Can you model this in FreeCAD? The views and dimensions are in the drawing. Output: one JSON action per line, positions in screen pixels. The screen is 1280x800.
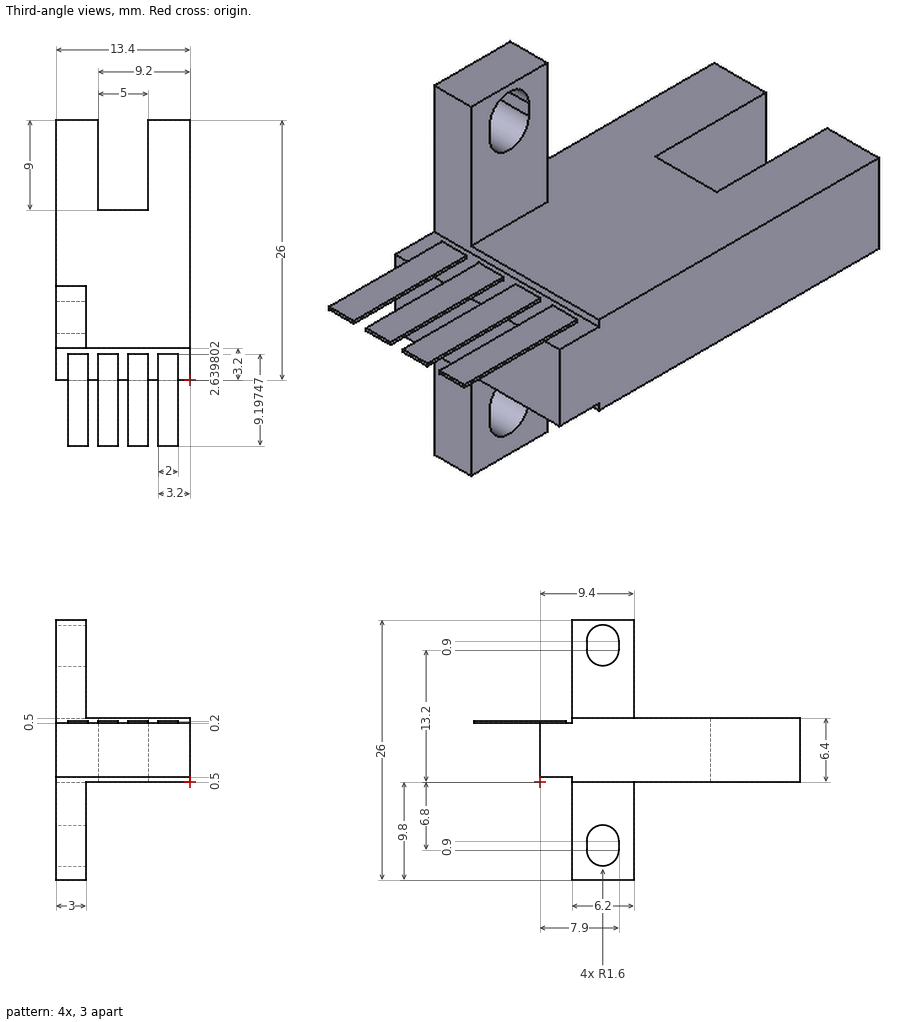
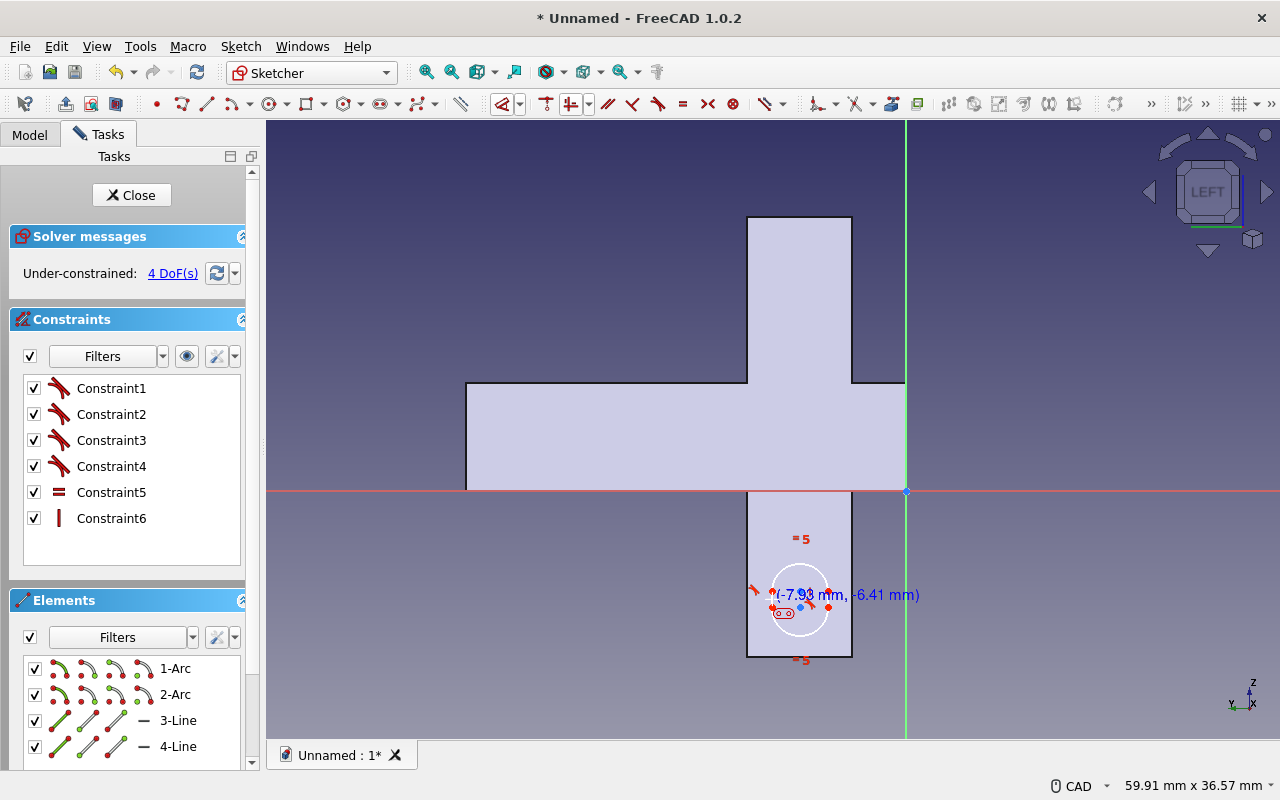
{"action": "left_click", "coordinate": [800, 268]}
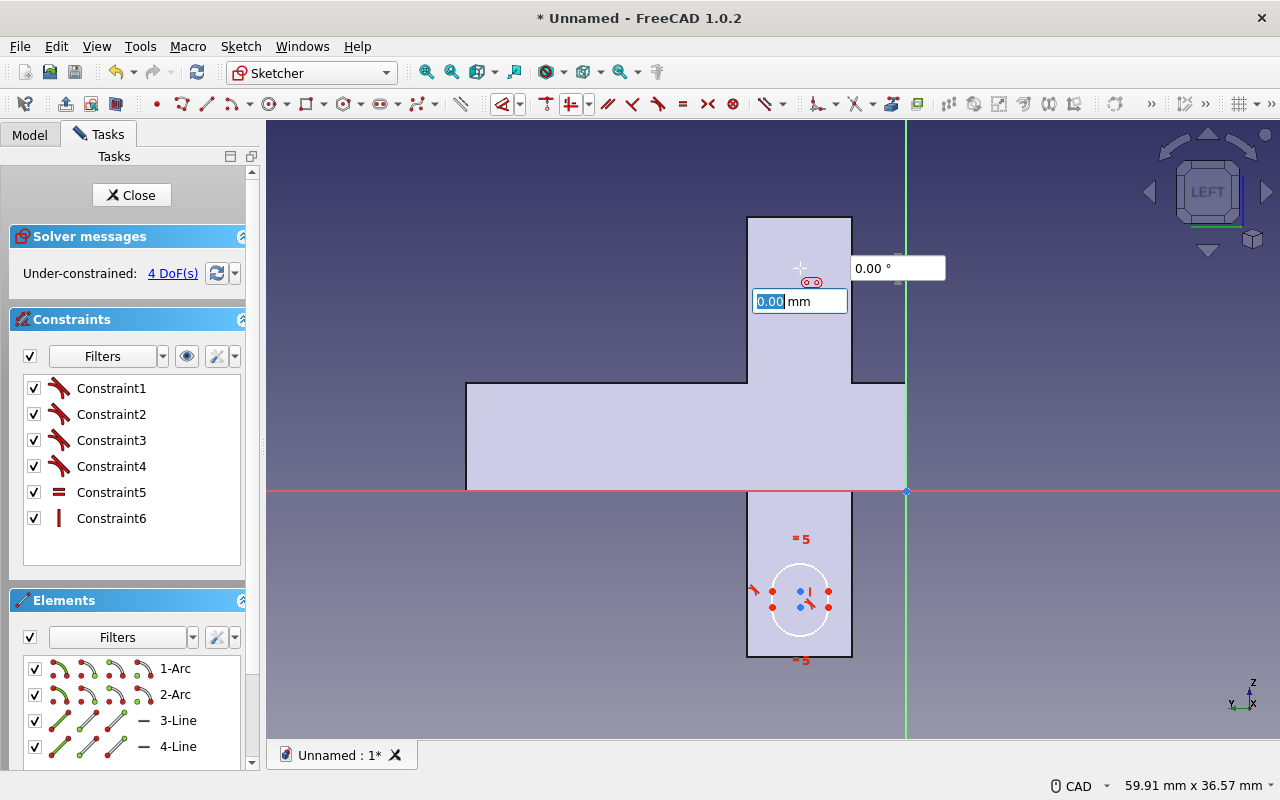
{"action": "left_click", "coordinate": [800, 253]}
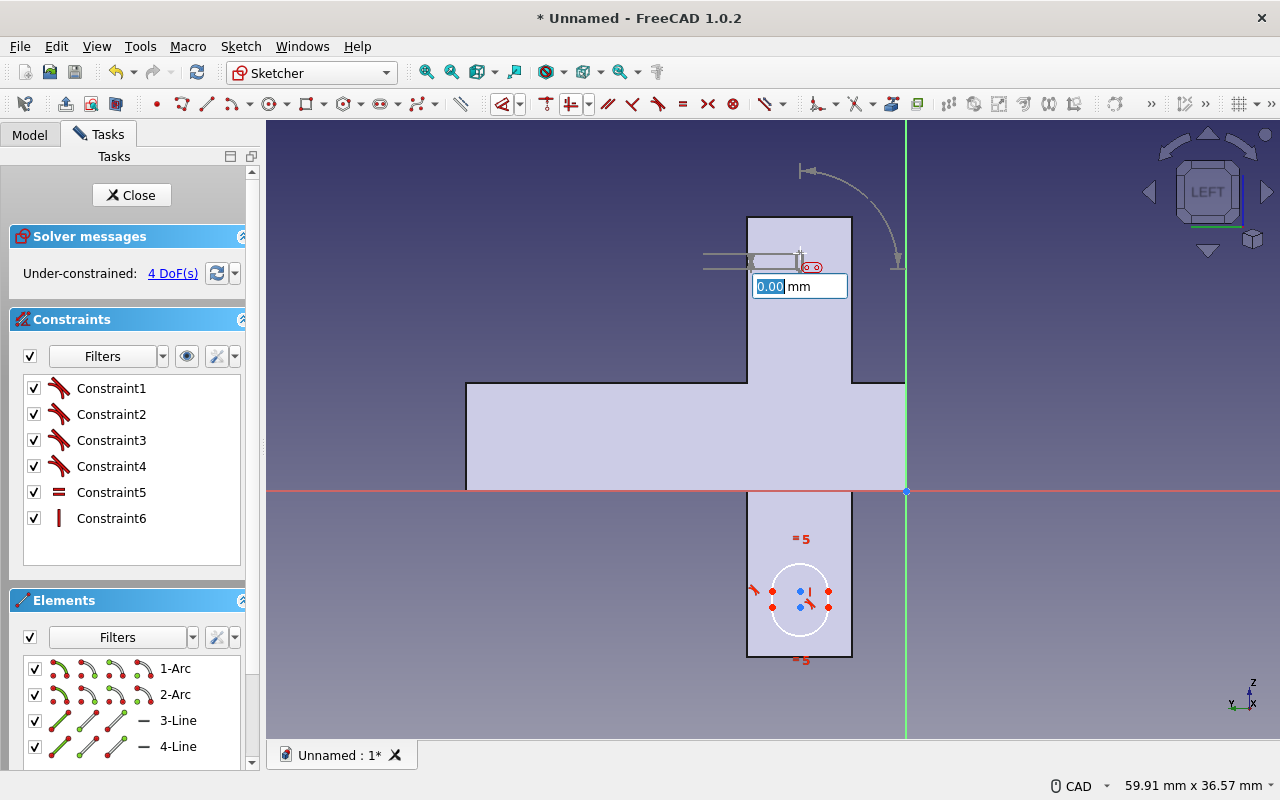
{"action": "left_click", "coordinate": [772, 260]}
{"action": "key", "text": "Escape"}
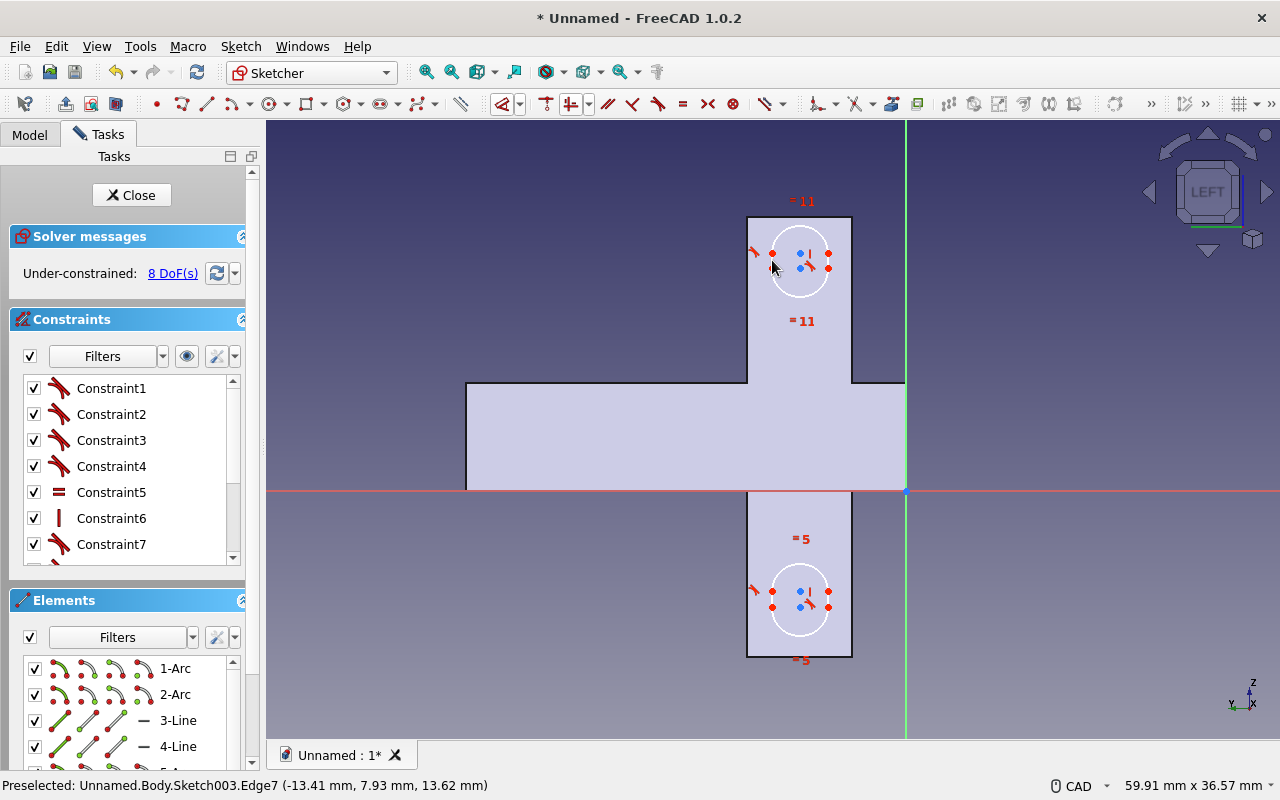
{"action": "left_click", "coordinate": [784, 631]}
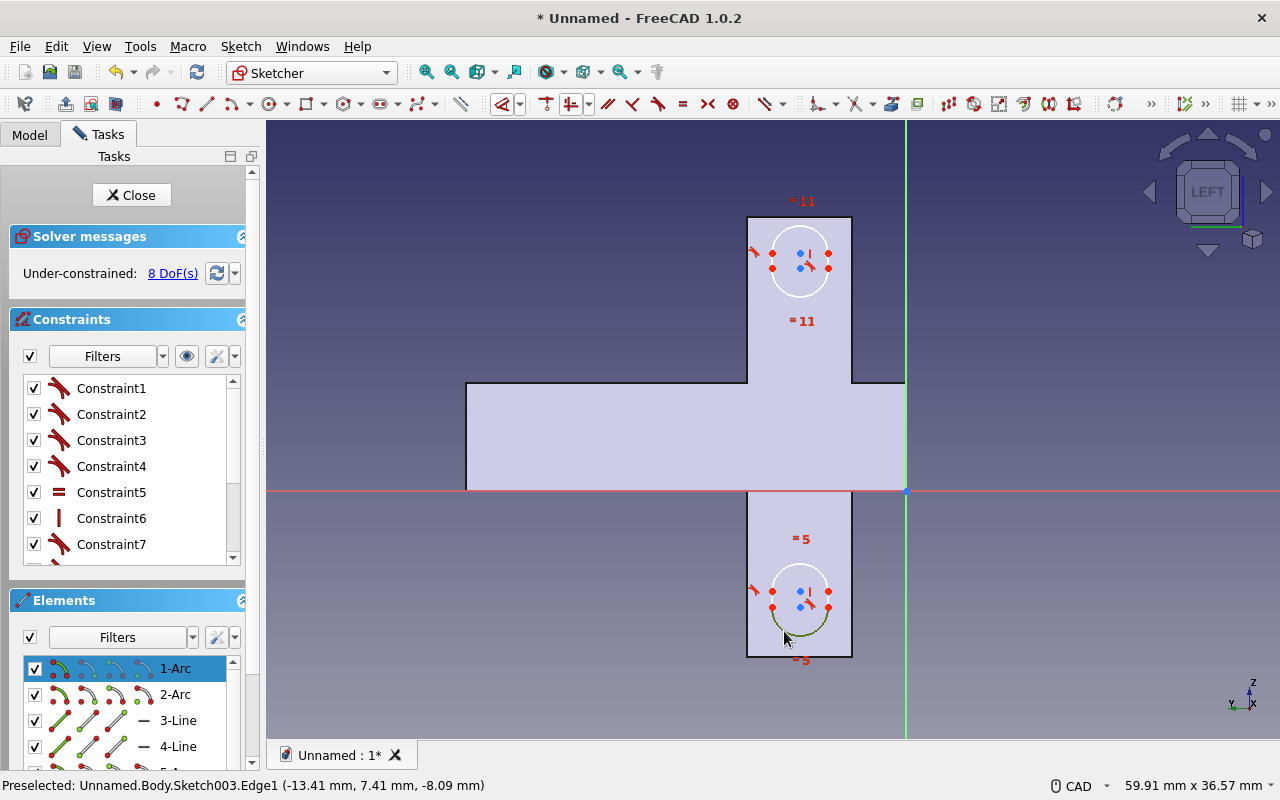
{"action": "left_click", "coordinate": [784, 292]}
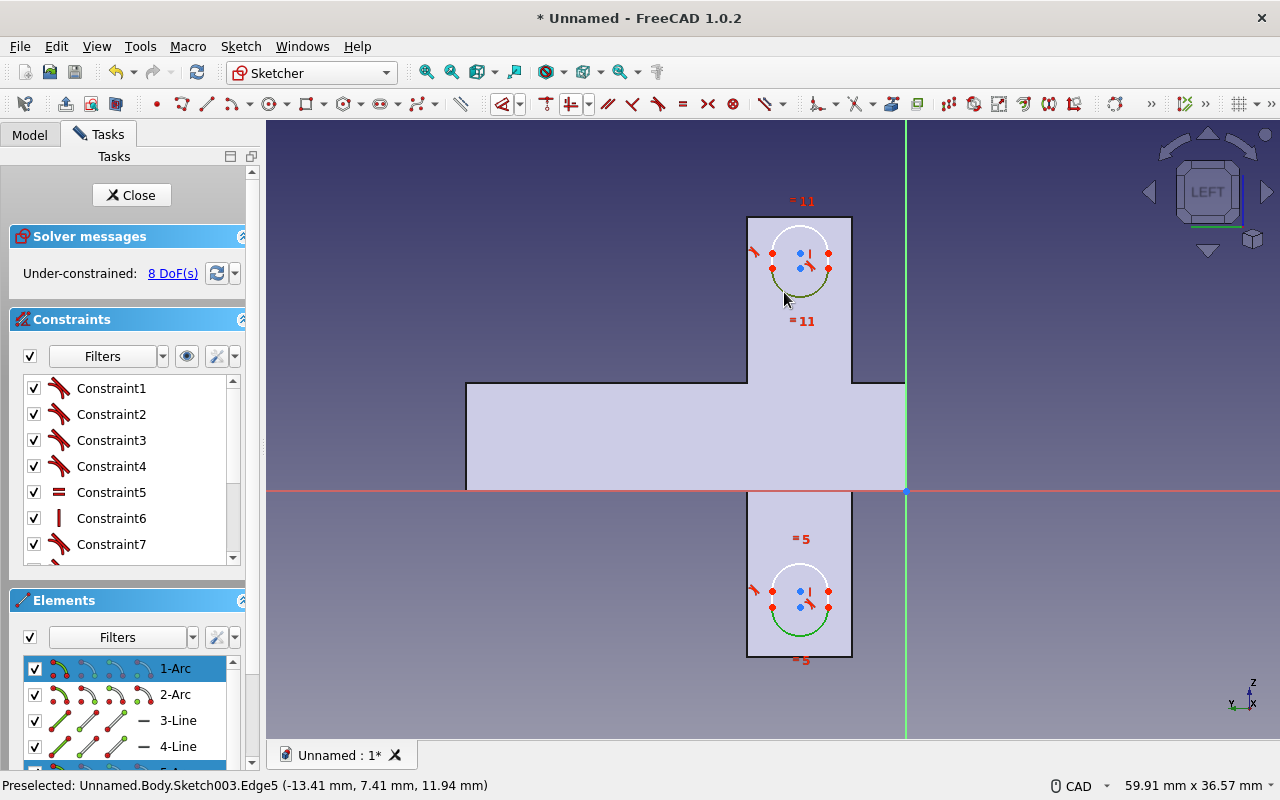
{"action": "left_click", "coordinate": [683, 104]}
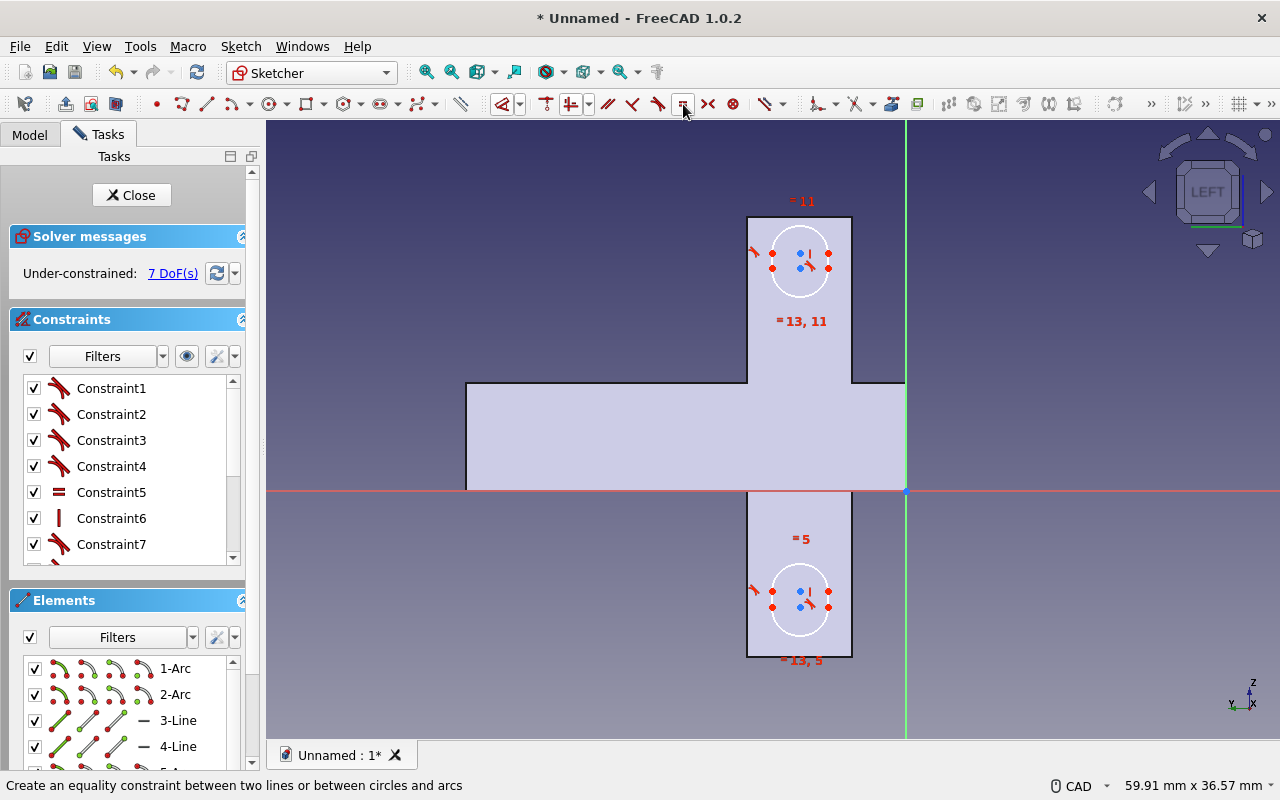
{"action": "scroll", "coordinate": [784, 631], "scroll_direction": "up", "scroll_amount": 2}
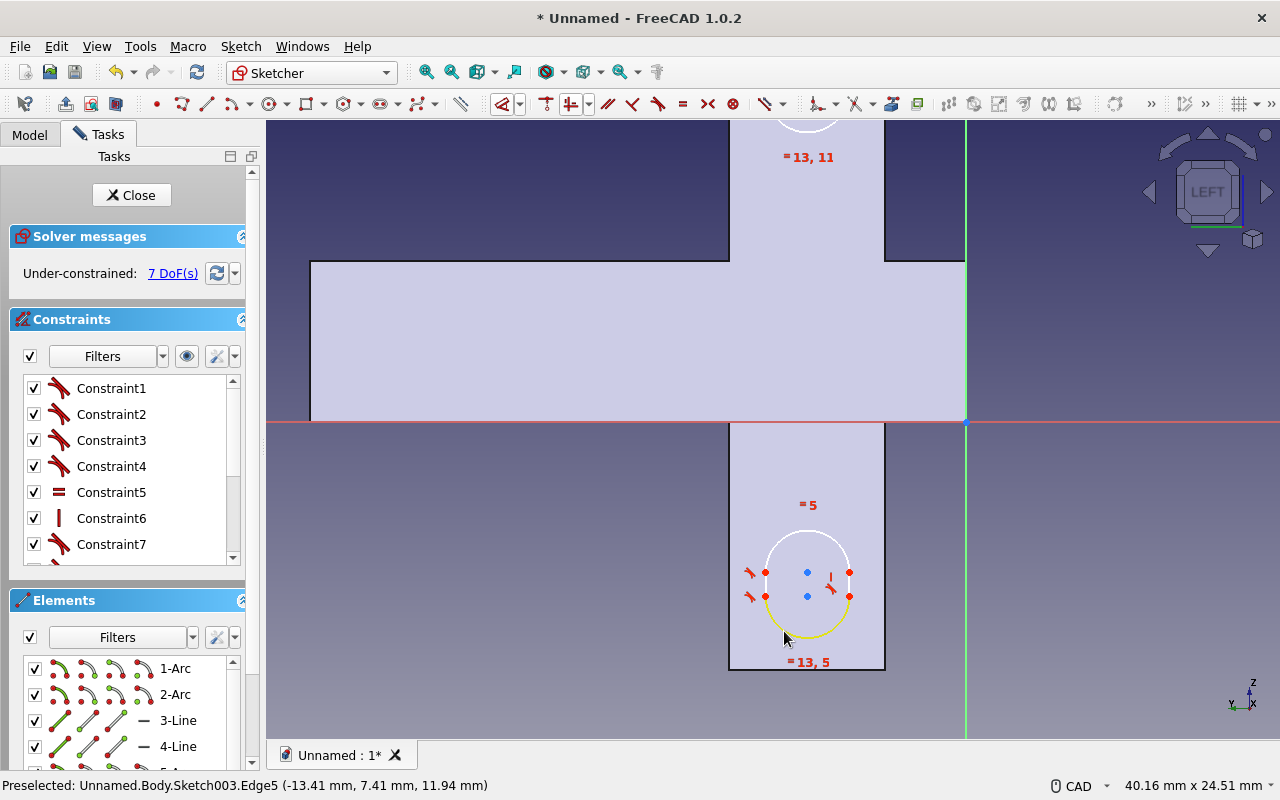
{"action": "left_click", "coordinate": [783, 630]}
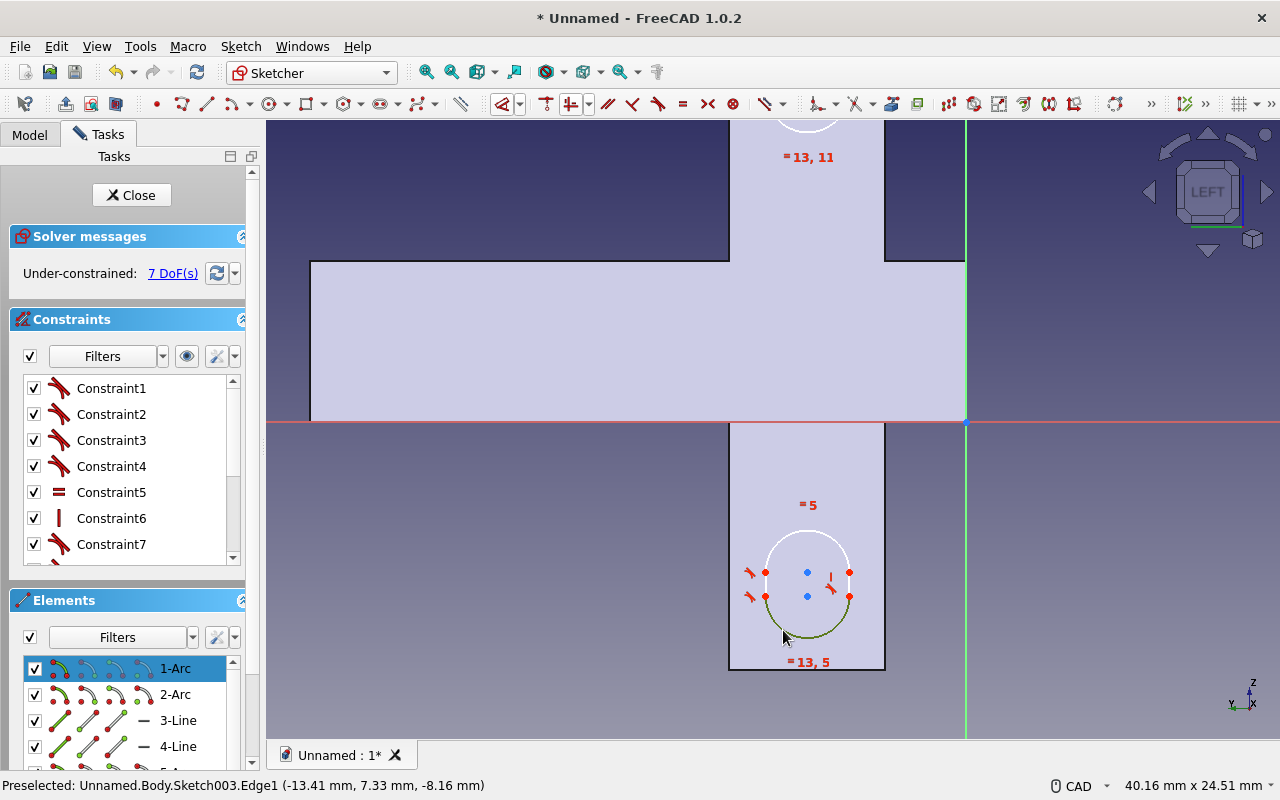
{"action": "left_click", "coordinate": [520, 104]}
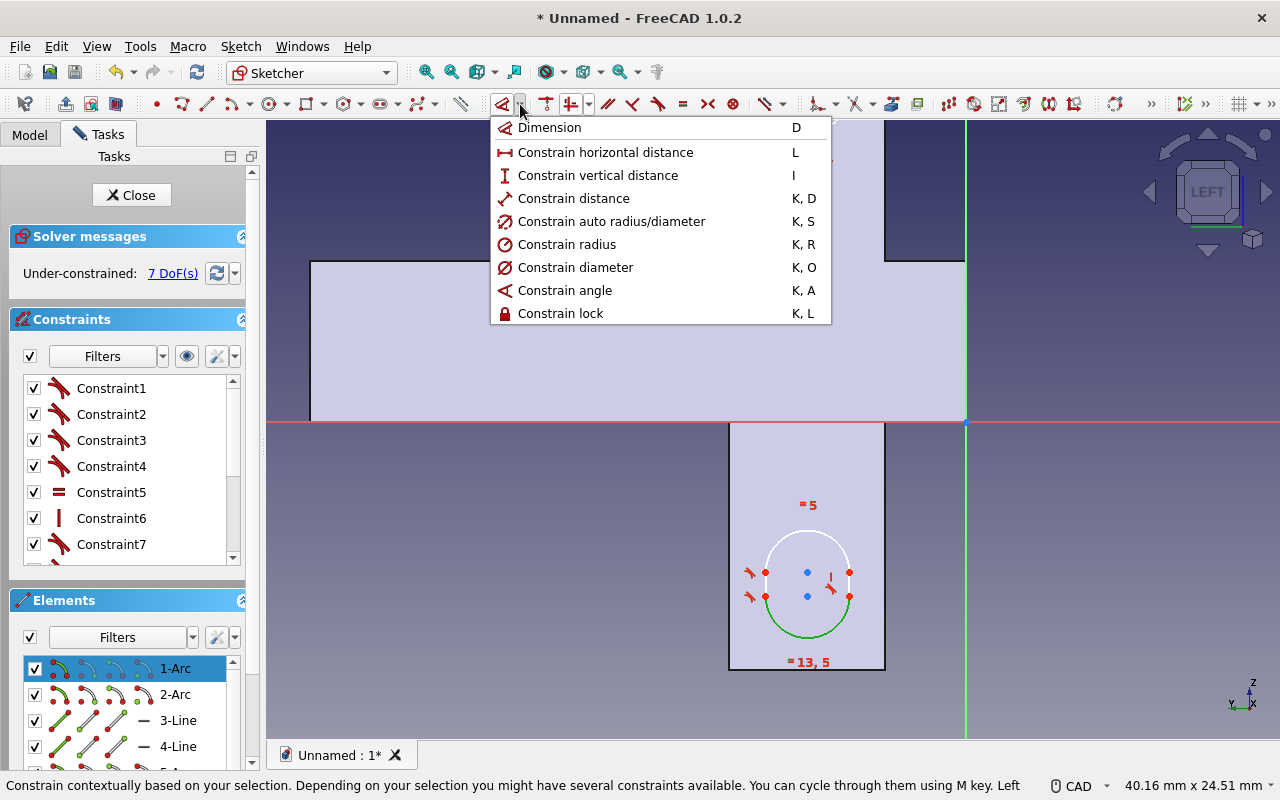
{"action": "left_click", "coordinate": [661, 244]}